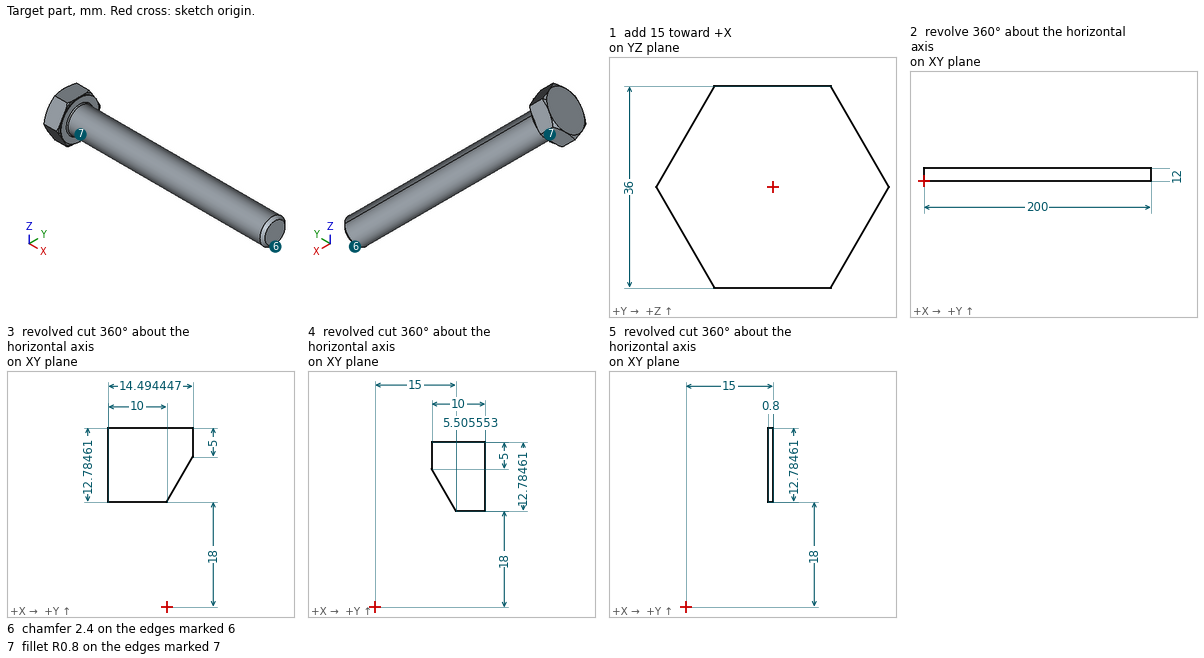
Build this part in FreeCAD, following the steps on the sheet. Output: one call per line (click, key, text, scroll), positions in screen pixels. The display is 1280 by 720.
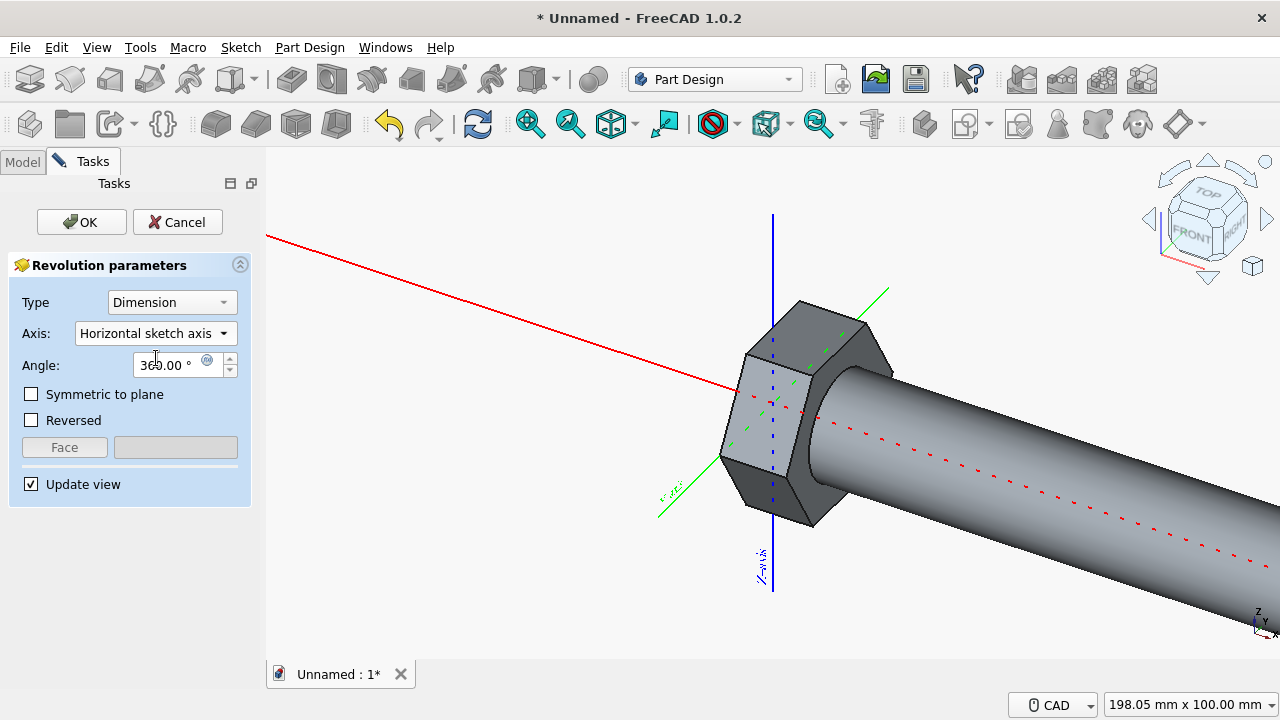
click(82, 222)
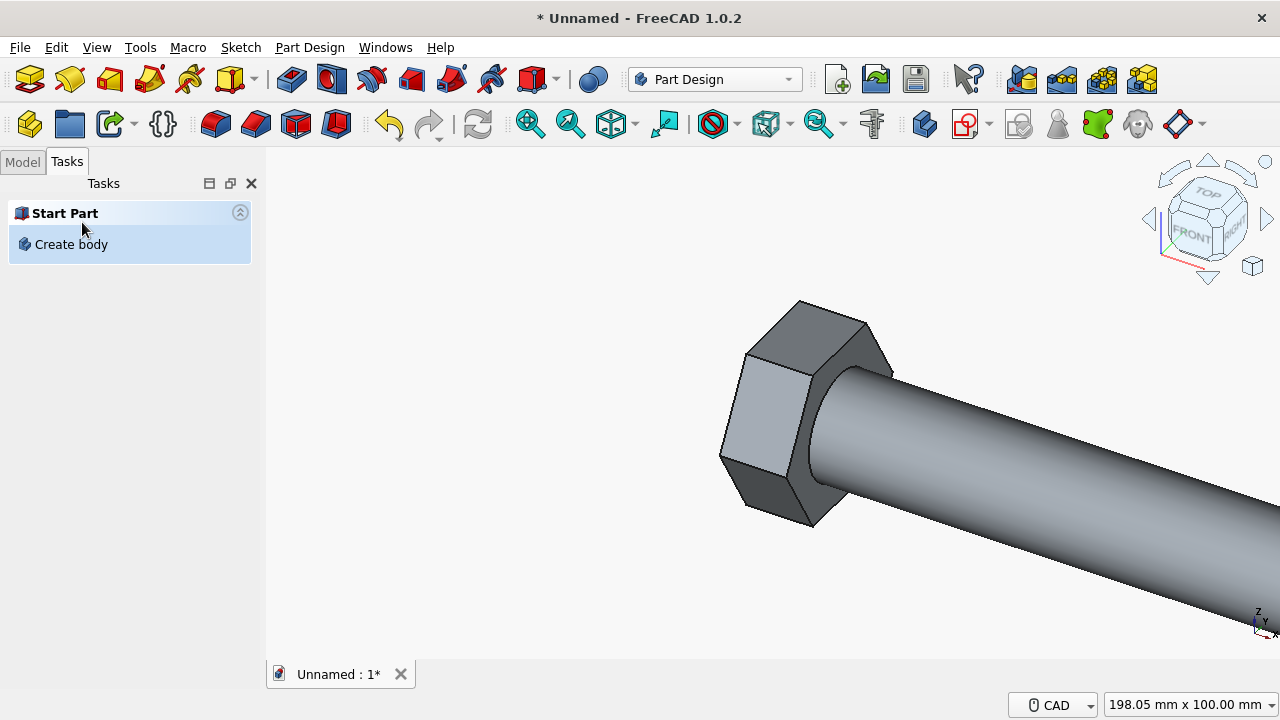
click(532, 124)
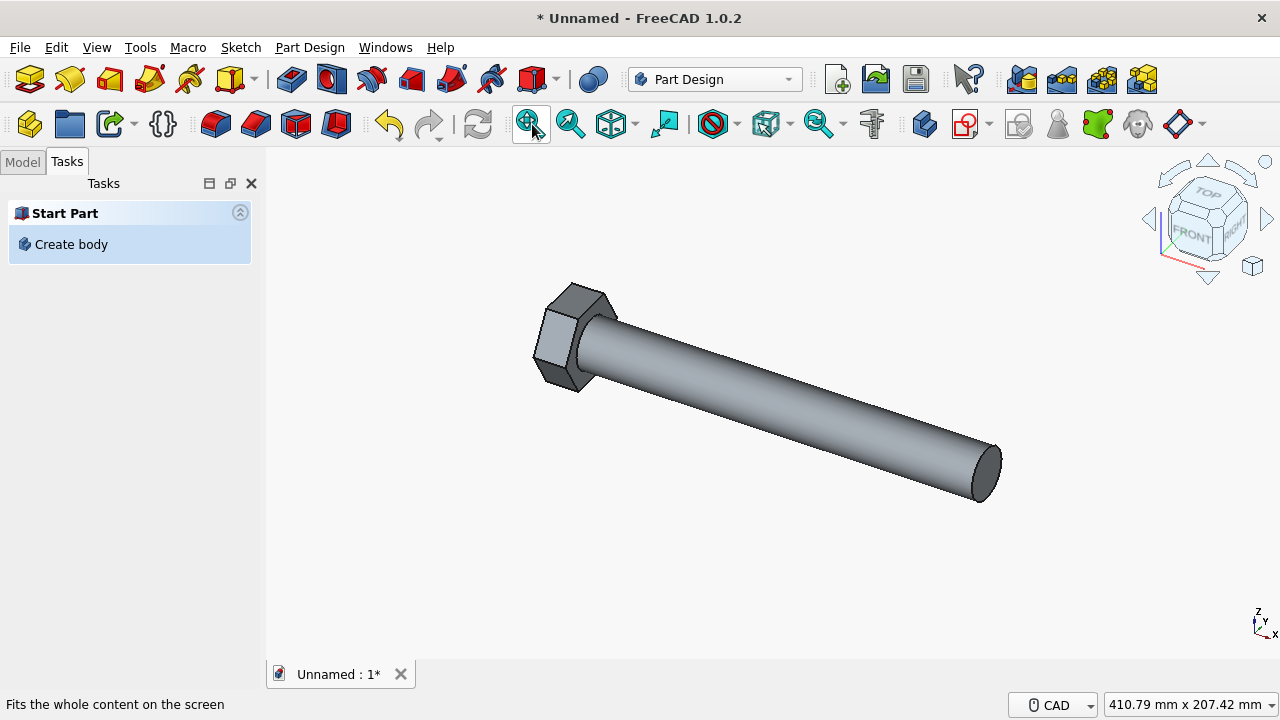
click(966, 124)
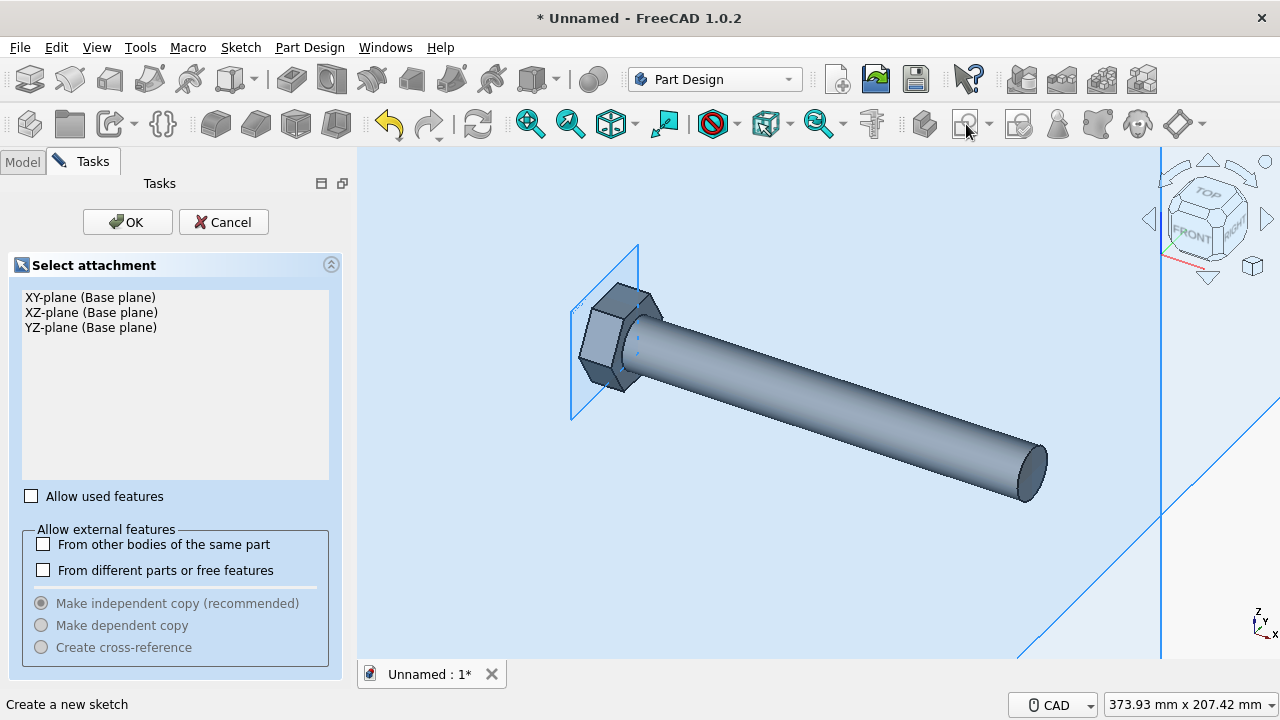
click(82, 298)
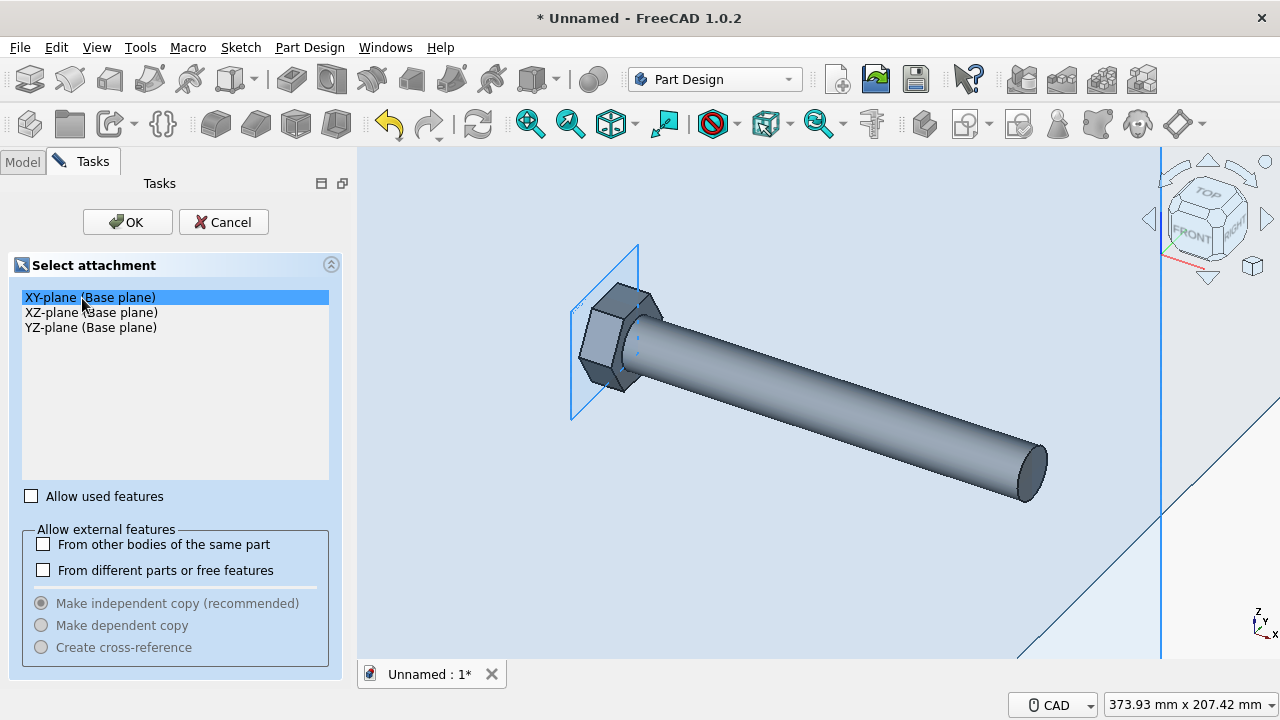
click(128, 222)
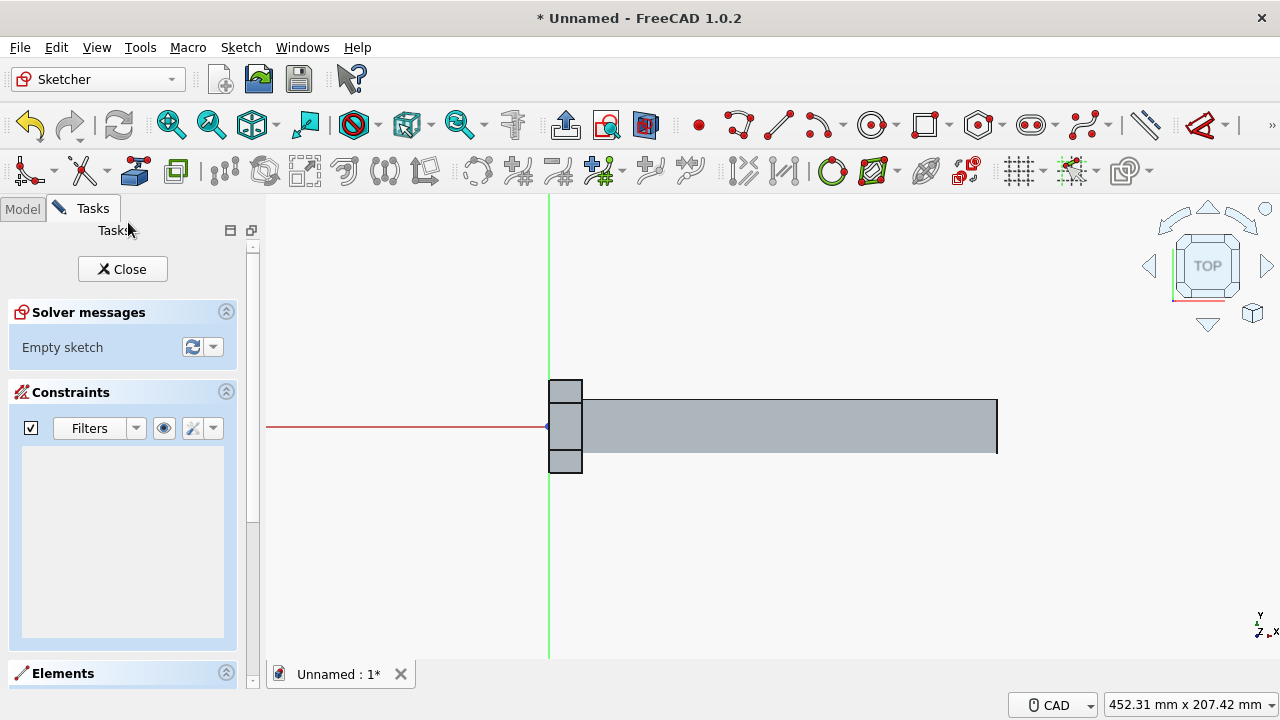
click(646, 126)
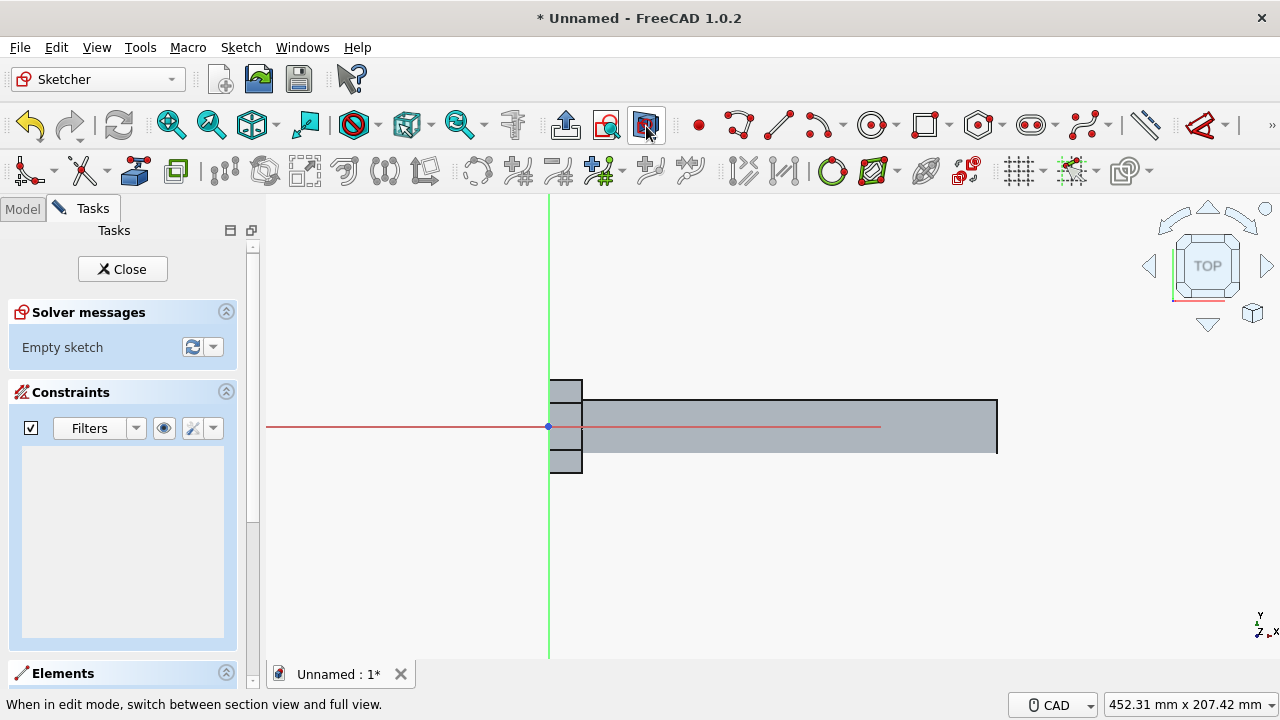
scroll(490, 381, up, 7)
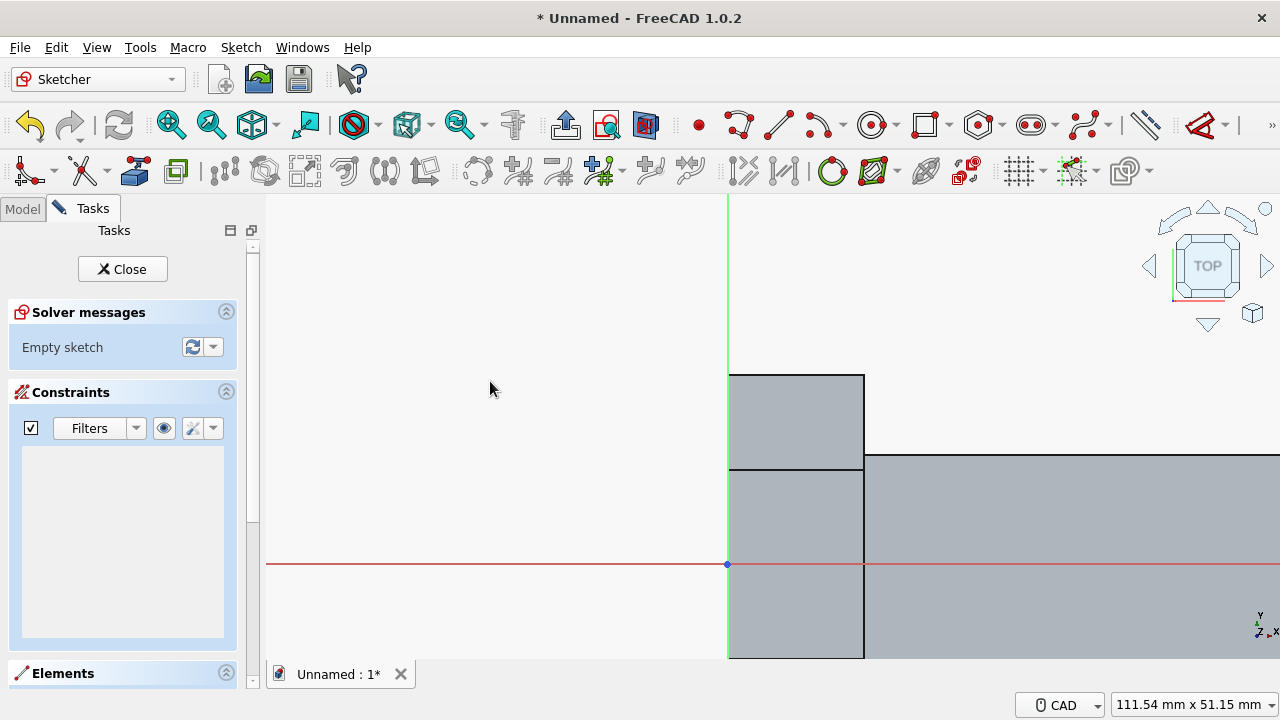
click(740, 126)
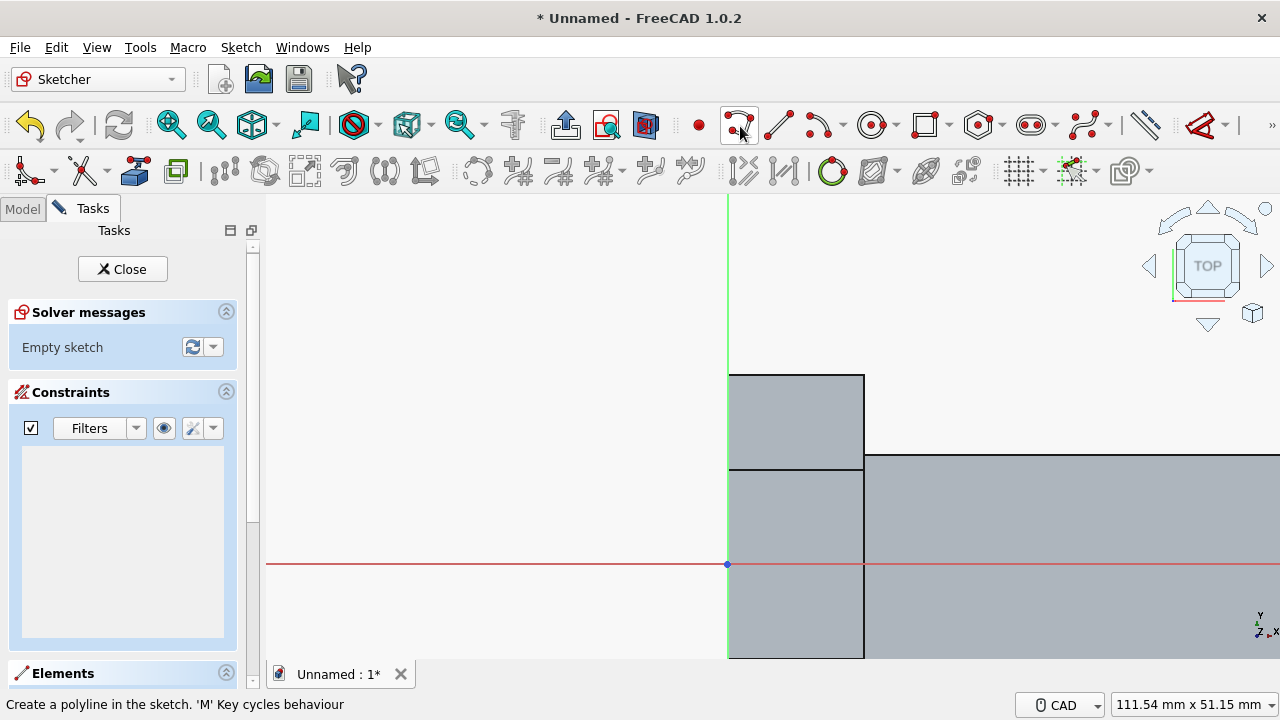
click(728, 401)
click(769, 330)
click(769, 284)
click(637, 284)
click(637, 401)
click(728, 402)
key(Escape)
key(Escape)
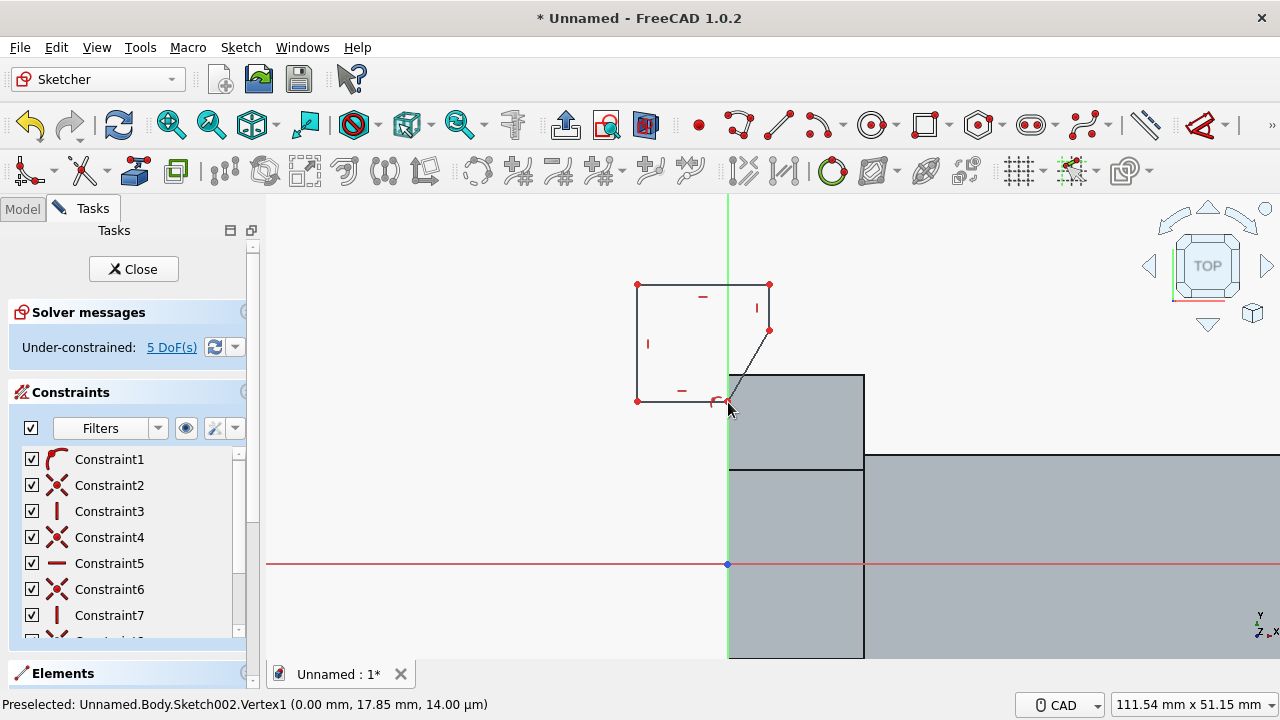
key(d)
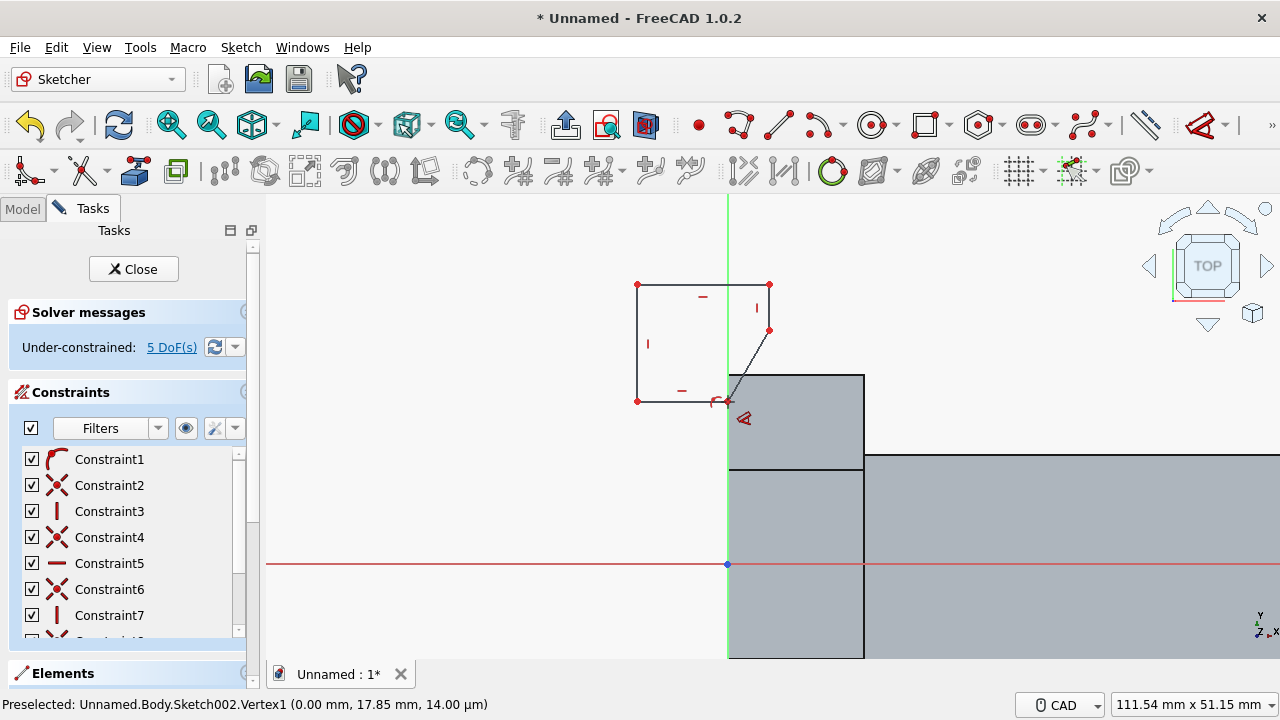
click(769, 317)
click(803, 308)